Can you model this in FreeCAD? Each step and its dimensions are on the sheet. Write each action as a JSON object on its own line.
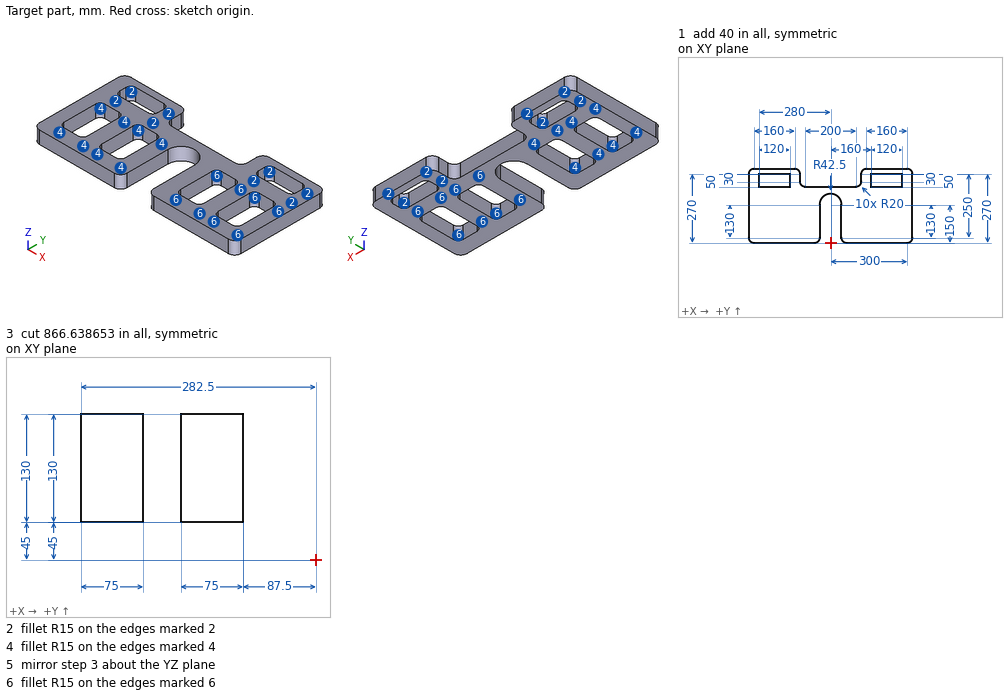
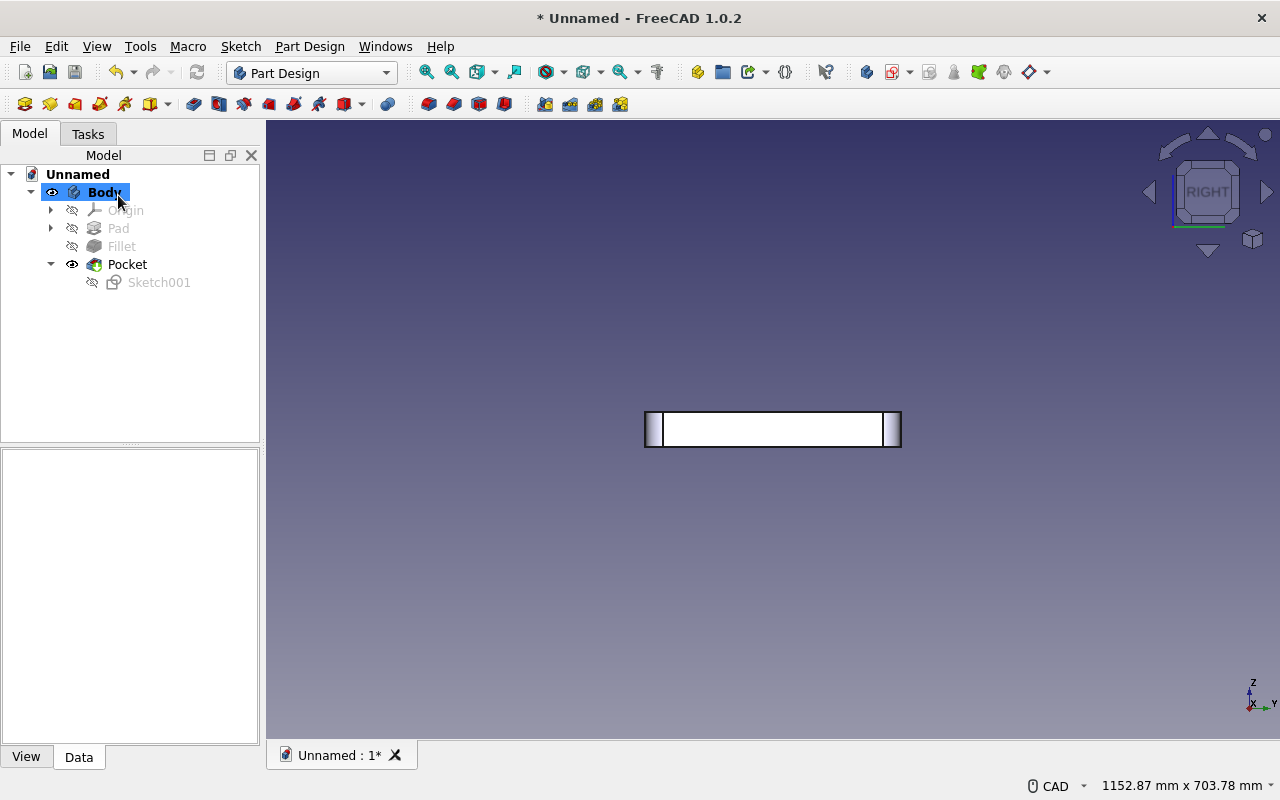
{"action": "key", "text": "v f"}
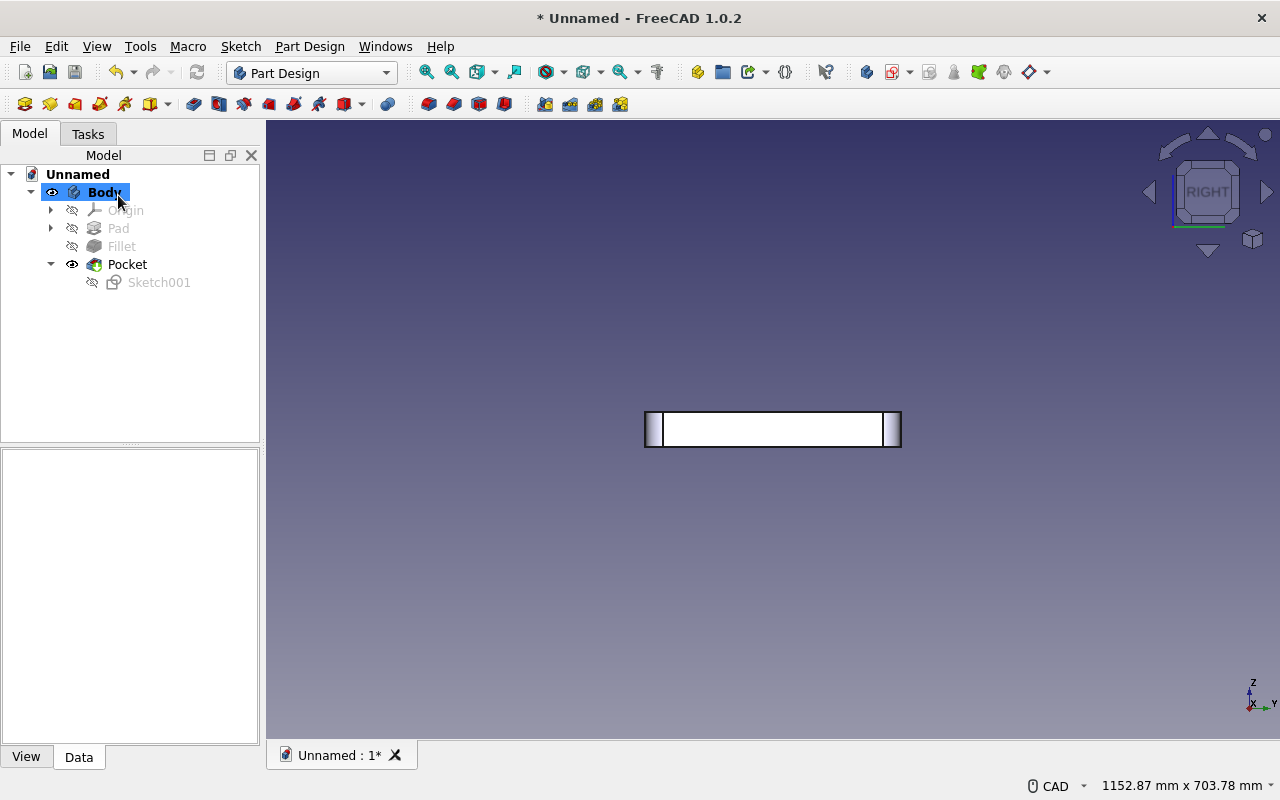
{"action": "key", "text": "5"}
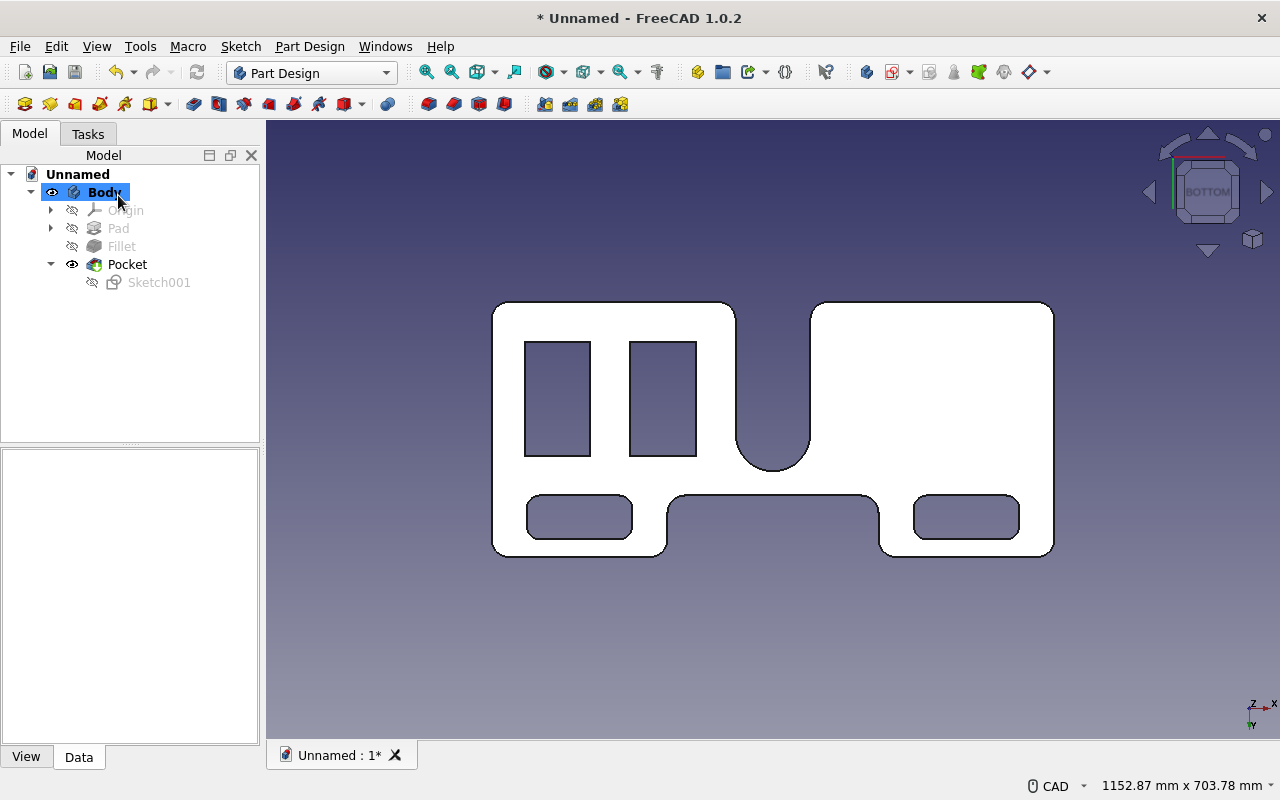
{"action": "key", "text": "4"}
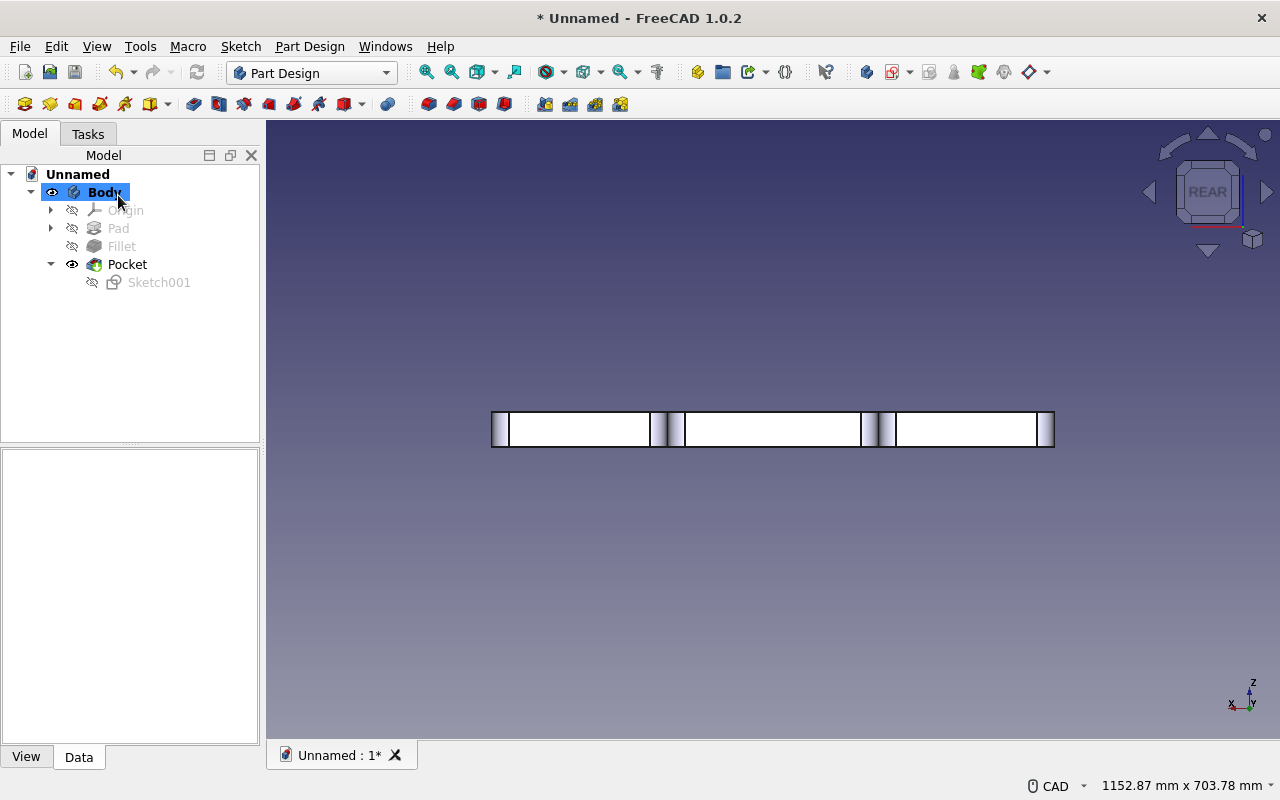
{"action": "key", "text": "6"}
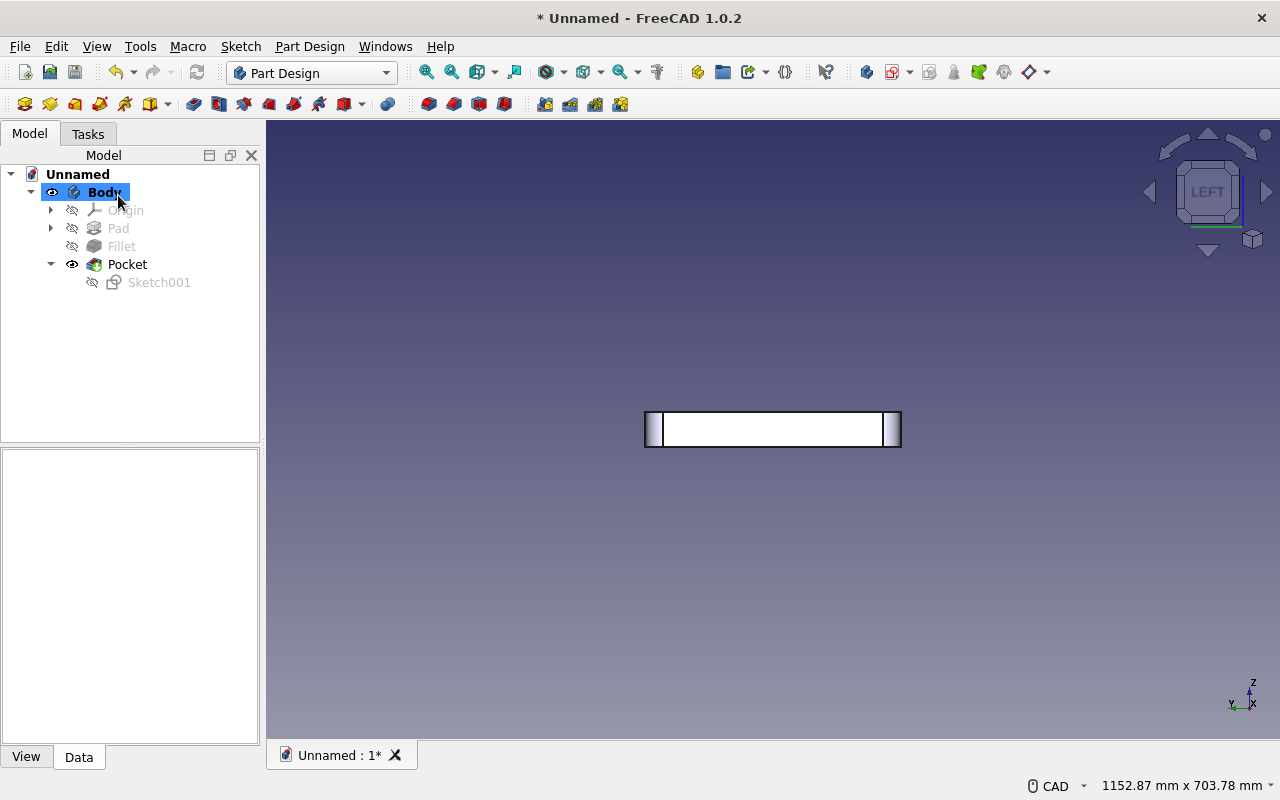
{"action": "key", "text": "v f"}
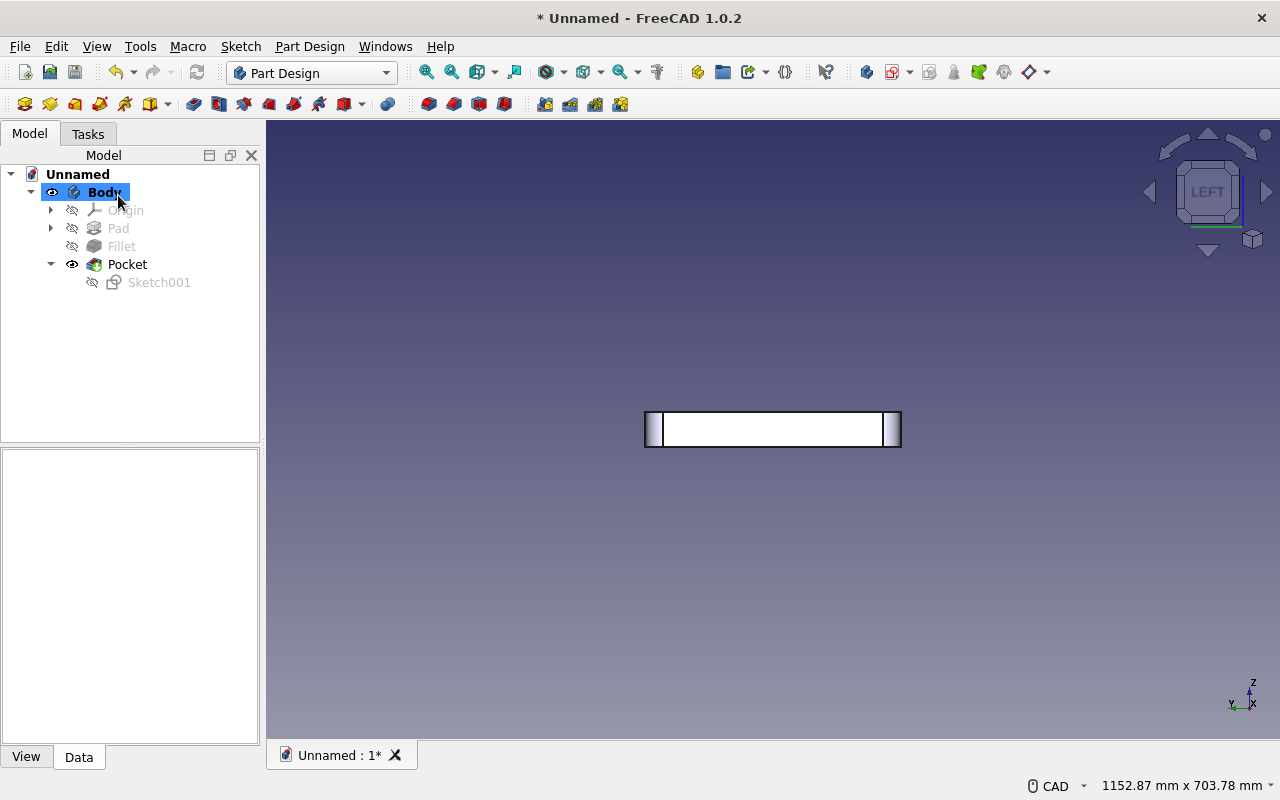
{"action": "key", "text": "v 3"}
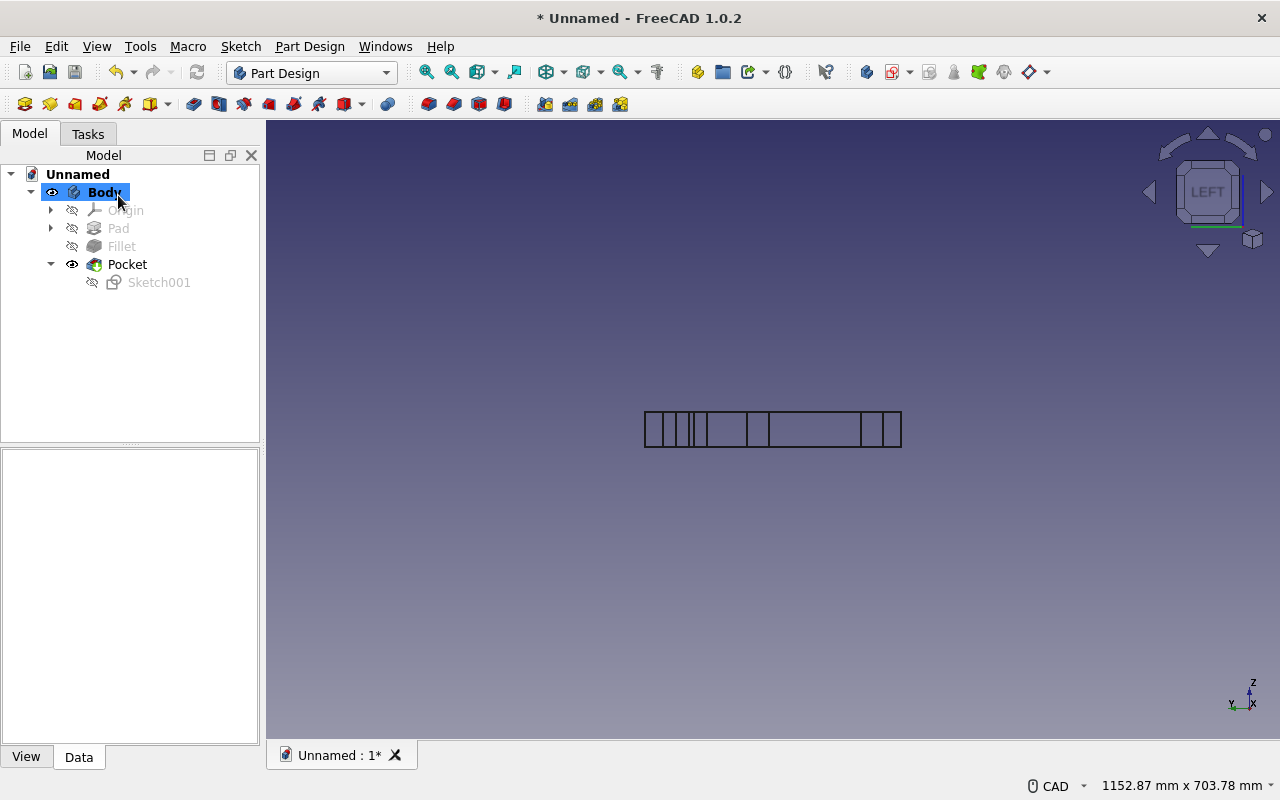
{"action": "key", "text": "0"}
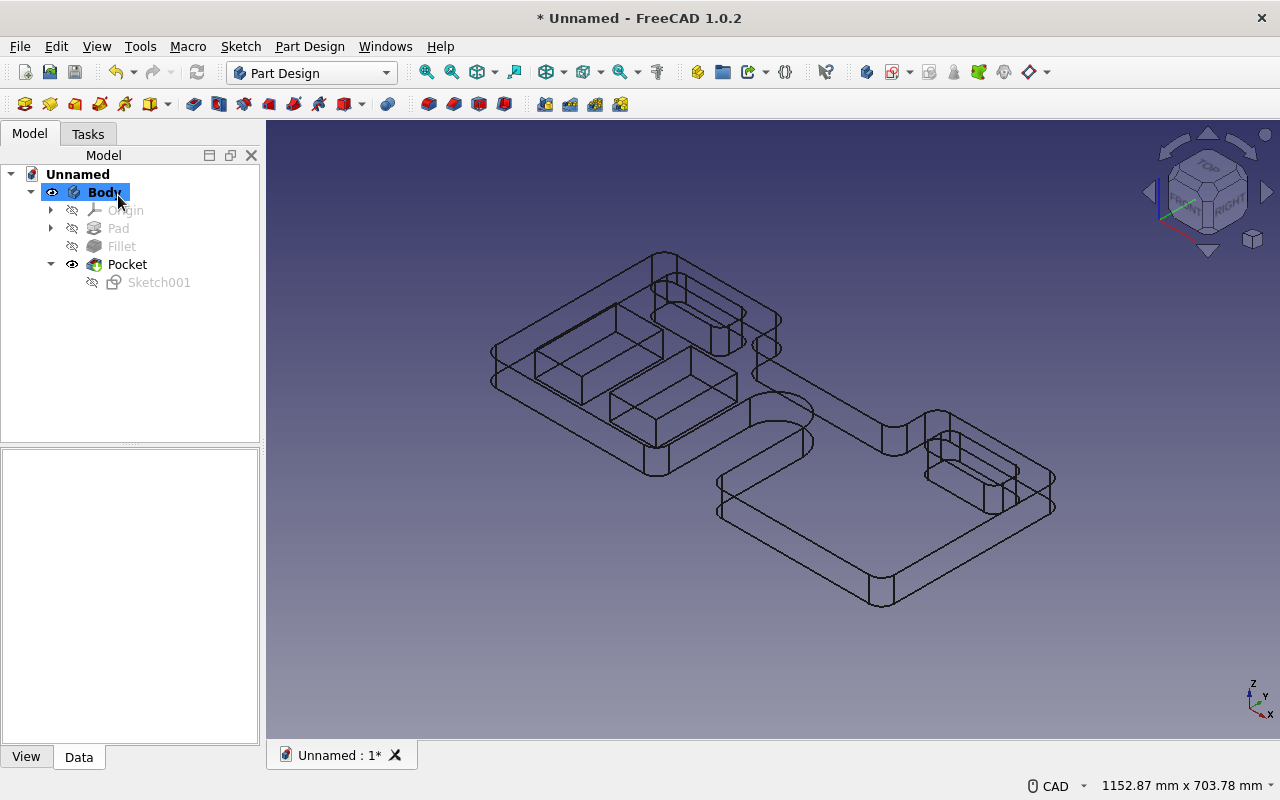
{"action": "left_click", "coordinate": [663, 343]}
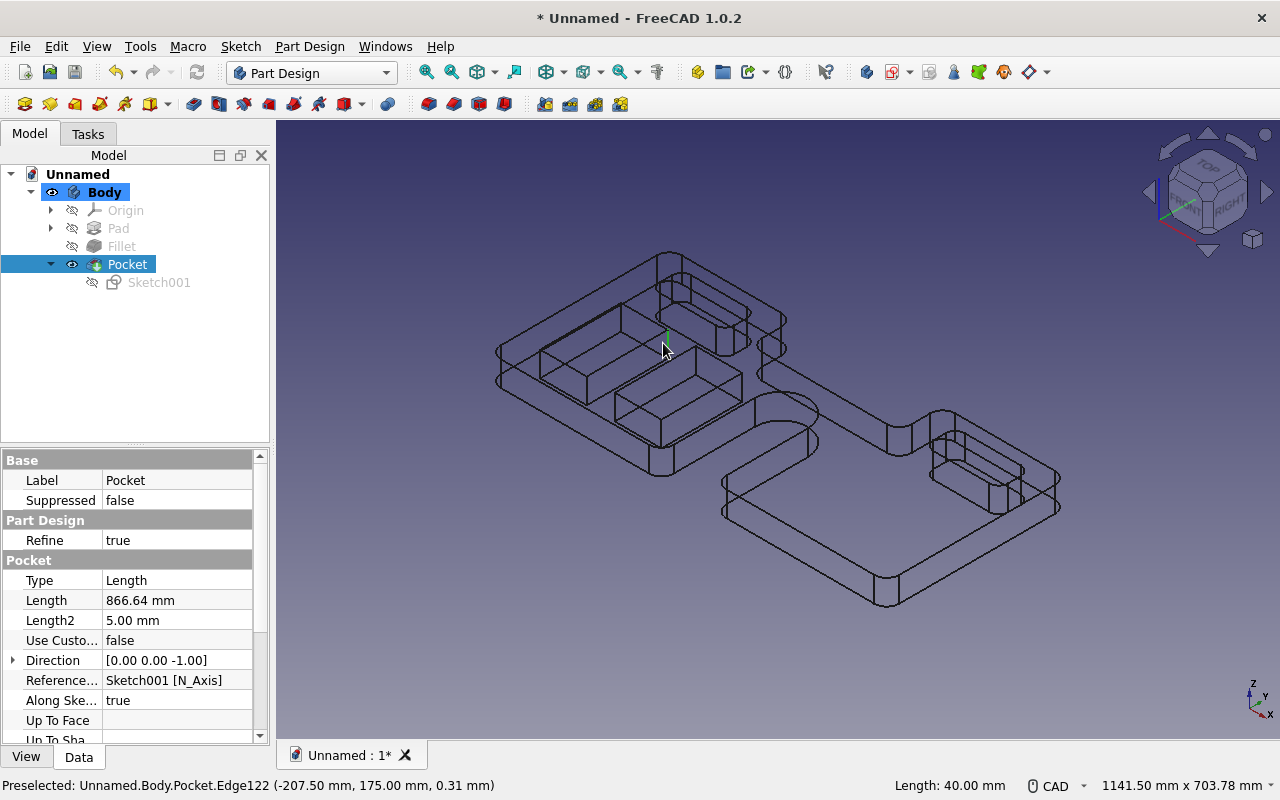
{"action": "left_click", "coordinate": [587, 390], "text": "ctrl"}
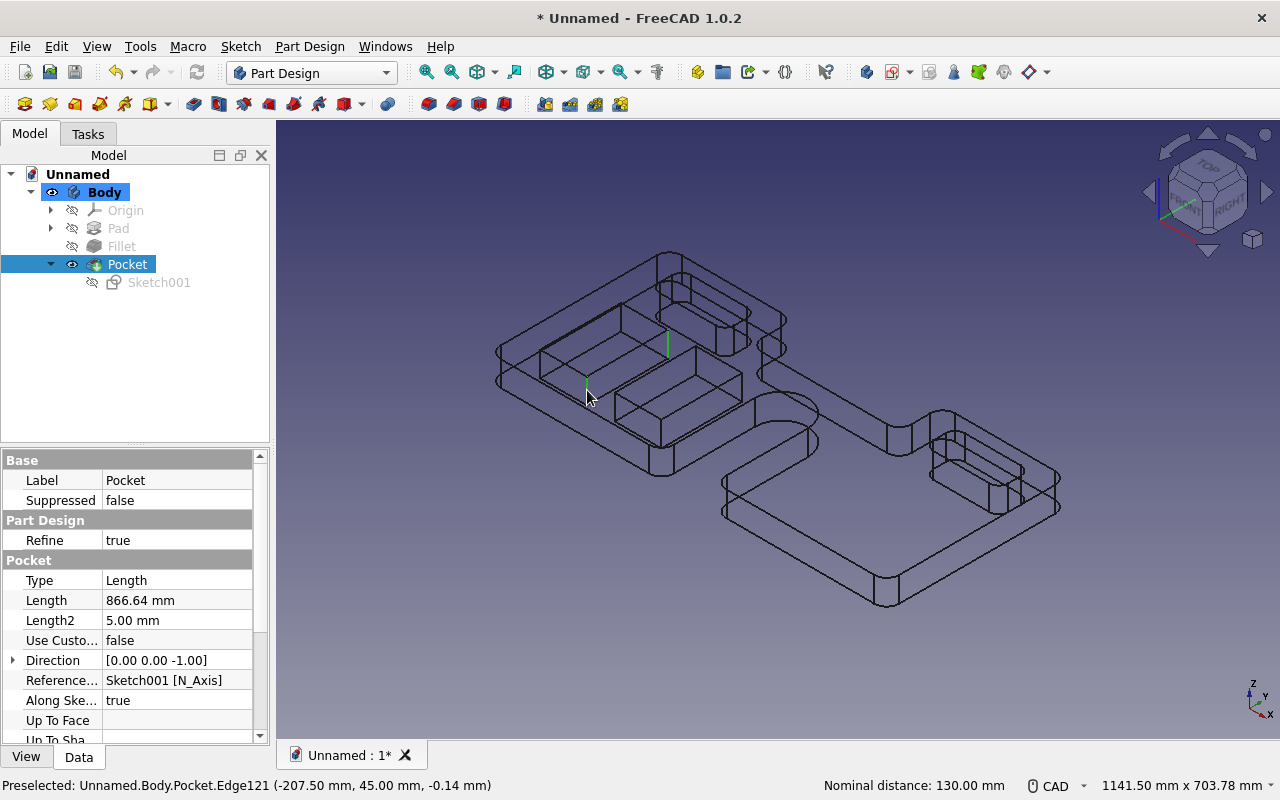
{"action": "left_click", "coordinate": [540, 363], "text": "ctrl"}